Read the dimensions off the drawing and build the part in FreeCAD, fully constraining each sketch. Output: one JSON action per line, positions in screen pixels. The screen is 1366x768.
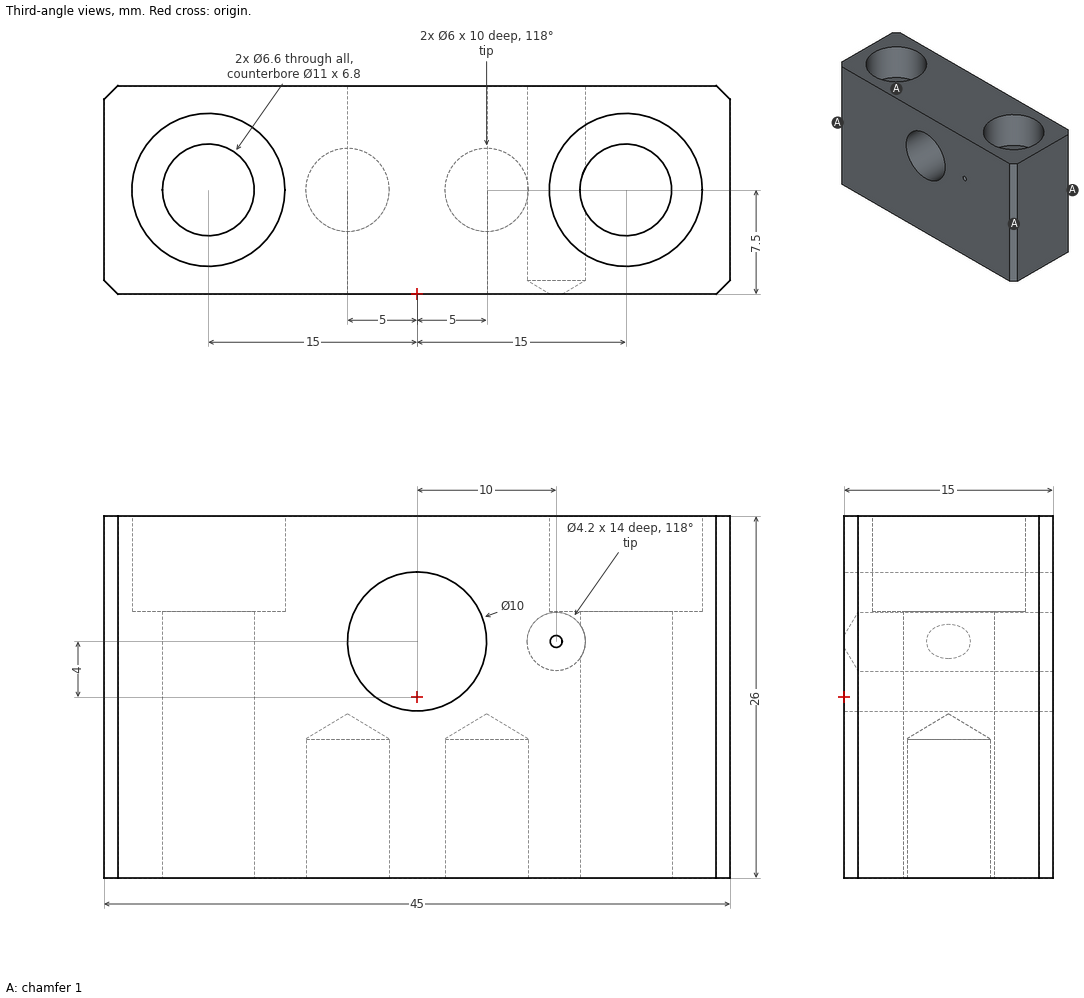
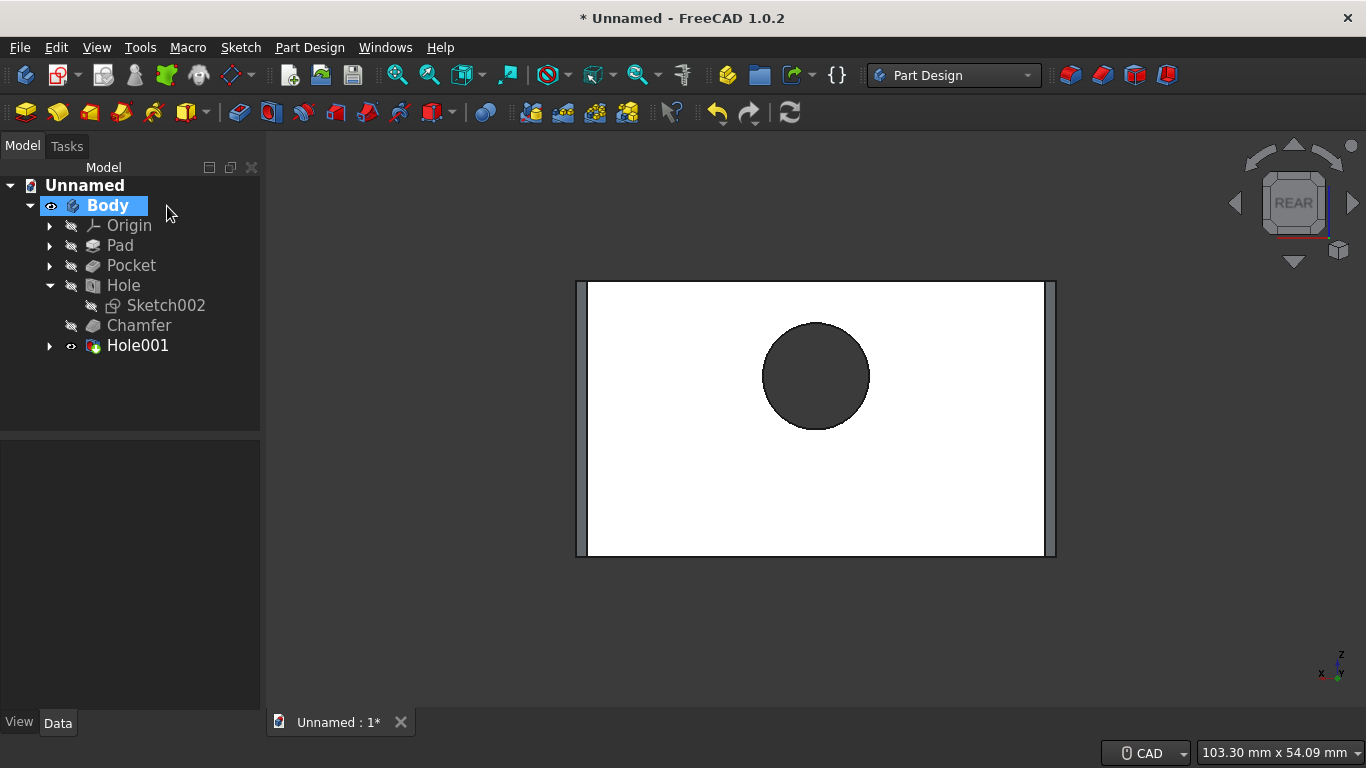
{"action": "left_click", "coordinate": [685, 458]}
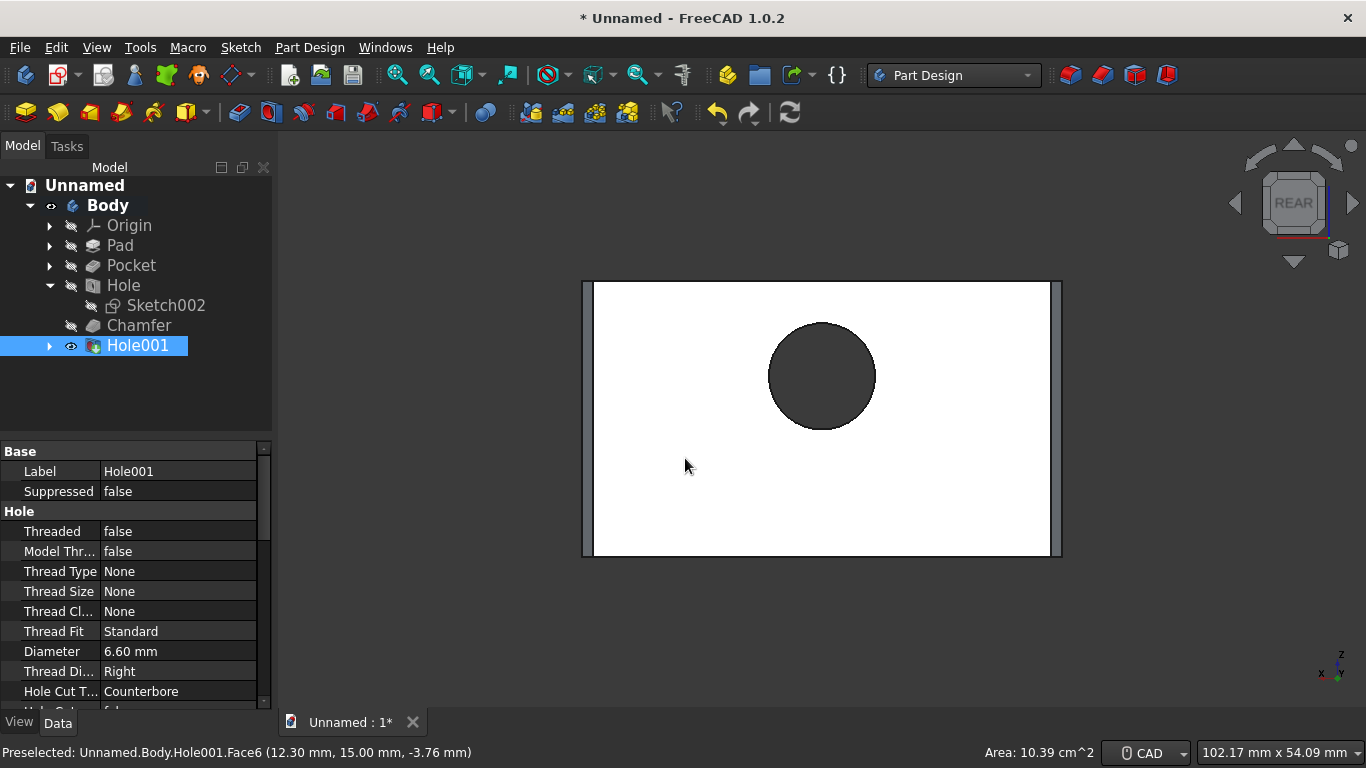
{"action": "left_click", "coordinate": [58, 76]}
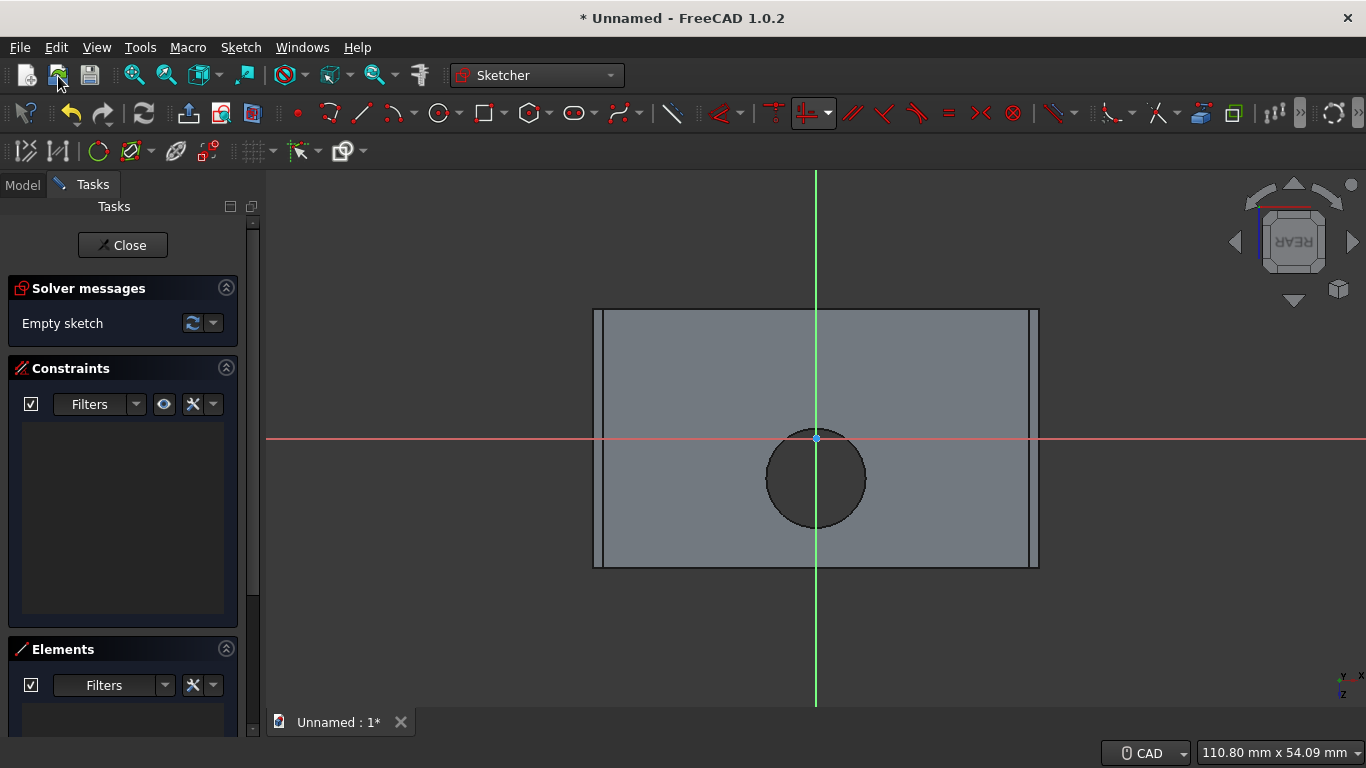
{"action": "scroll", "coordinate": [942, 484], "scroll_direction": "up", "scroll_amount": 10}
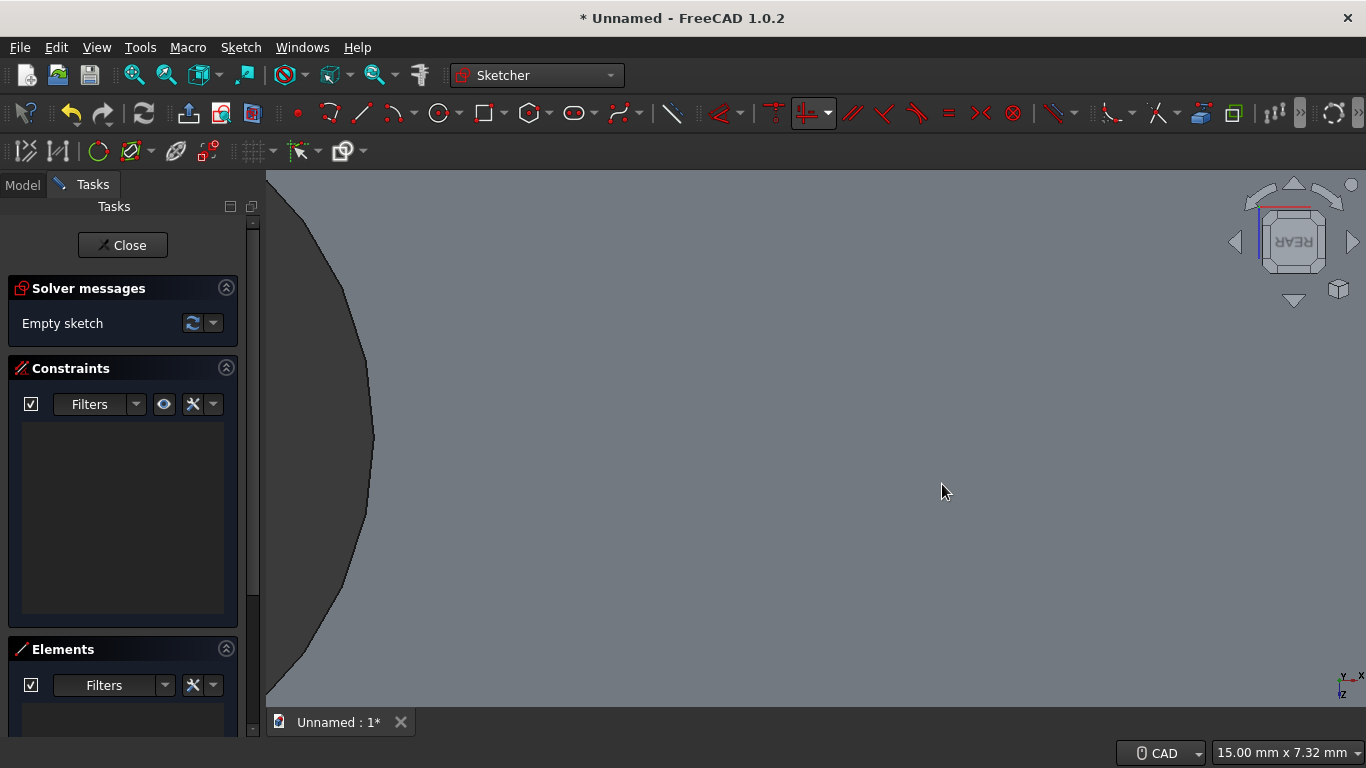
{"action": "left_click", "coordinate": [440, 114]}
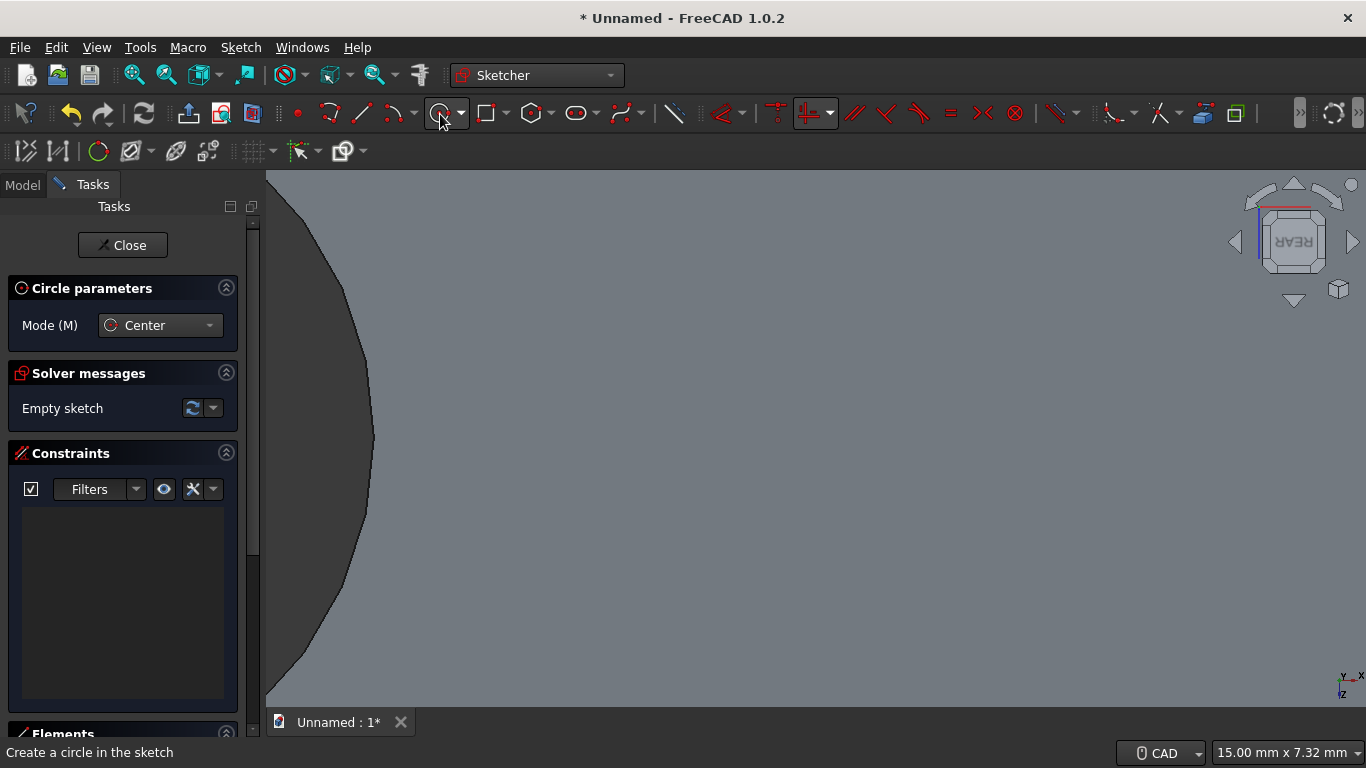
{"action": "left_click", "coordinate": [741, 437]}
{"action": "left_click", "coordinate": [850, 329]}
{"action": "key", "text": "Escape"}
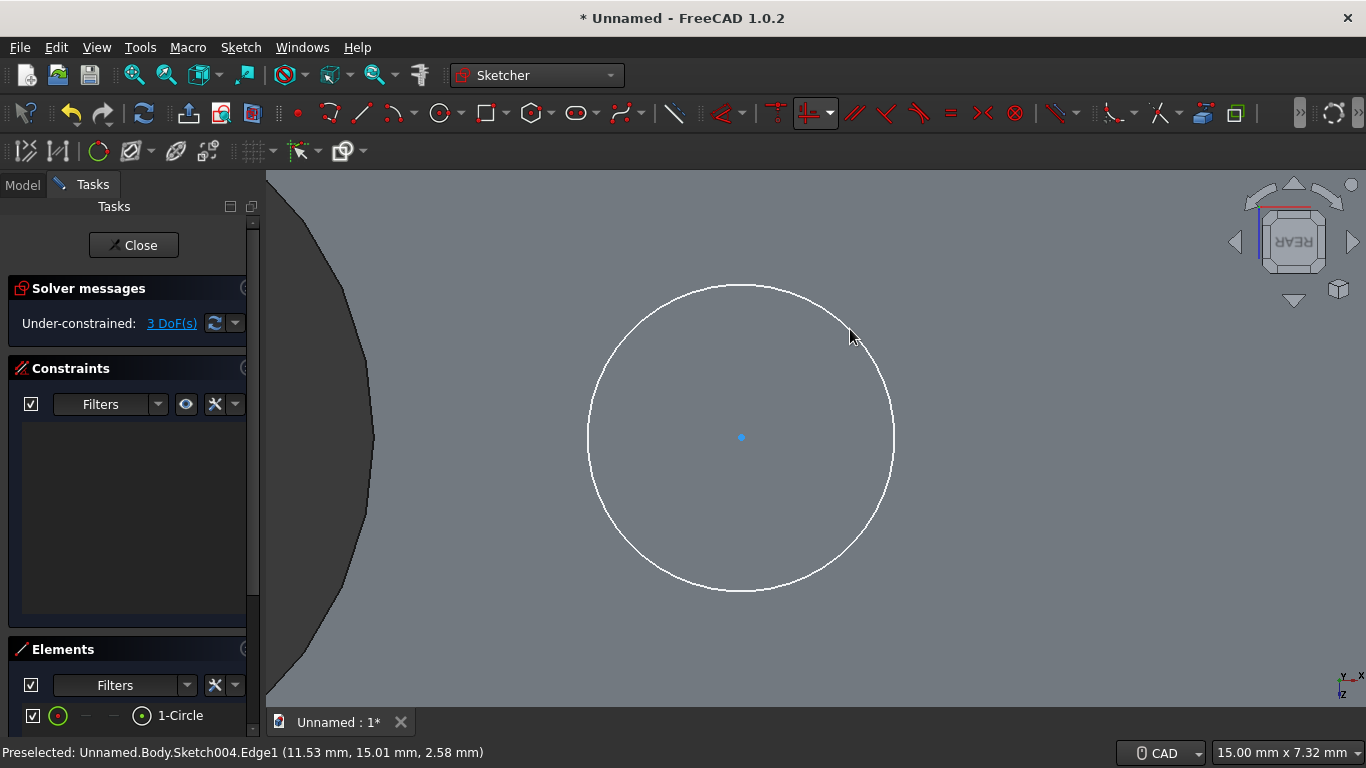
{"action": "left_click", "coordinate": [722, 114]}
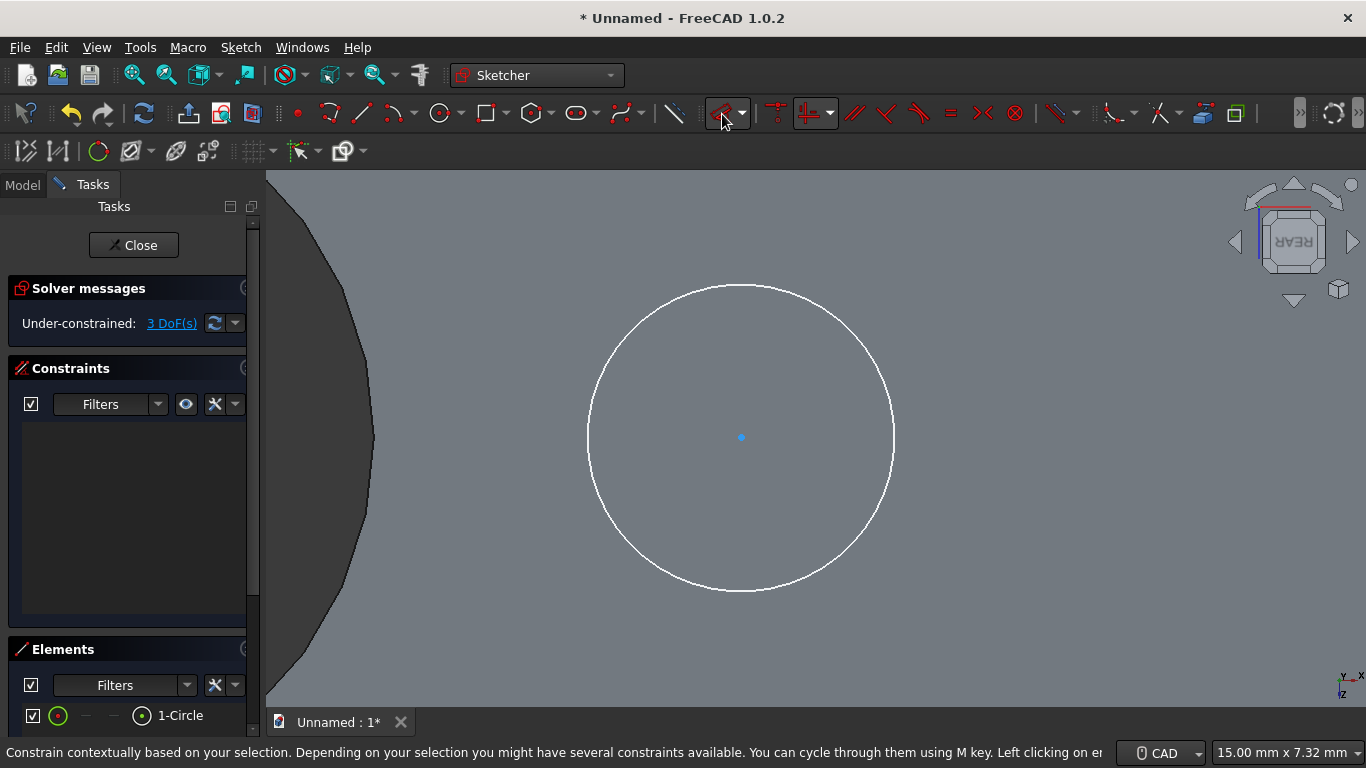
{"action": "left_click", "coordinate": [849, 329]}
{"action": "left_click", "coordinate": [872, 306]}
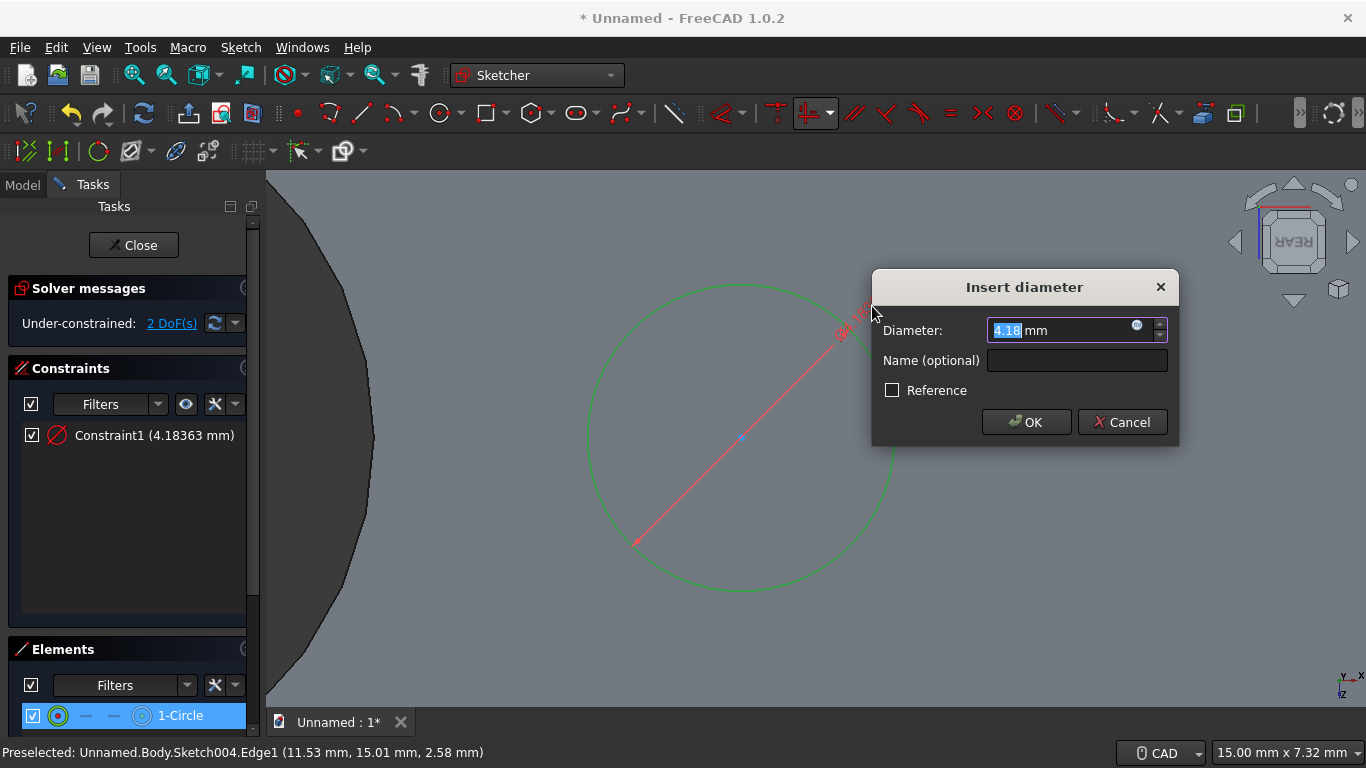
{"action": "type", "text": "4.2"}
{"action": "key", "text": "Return"}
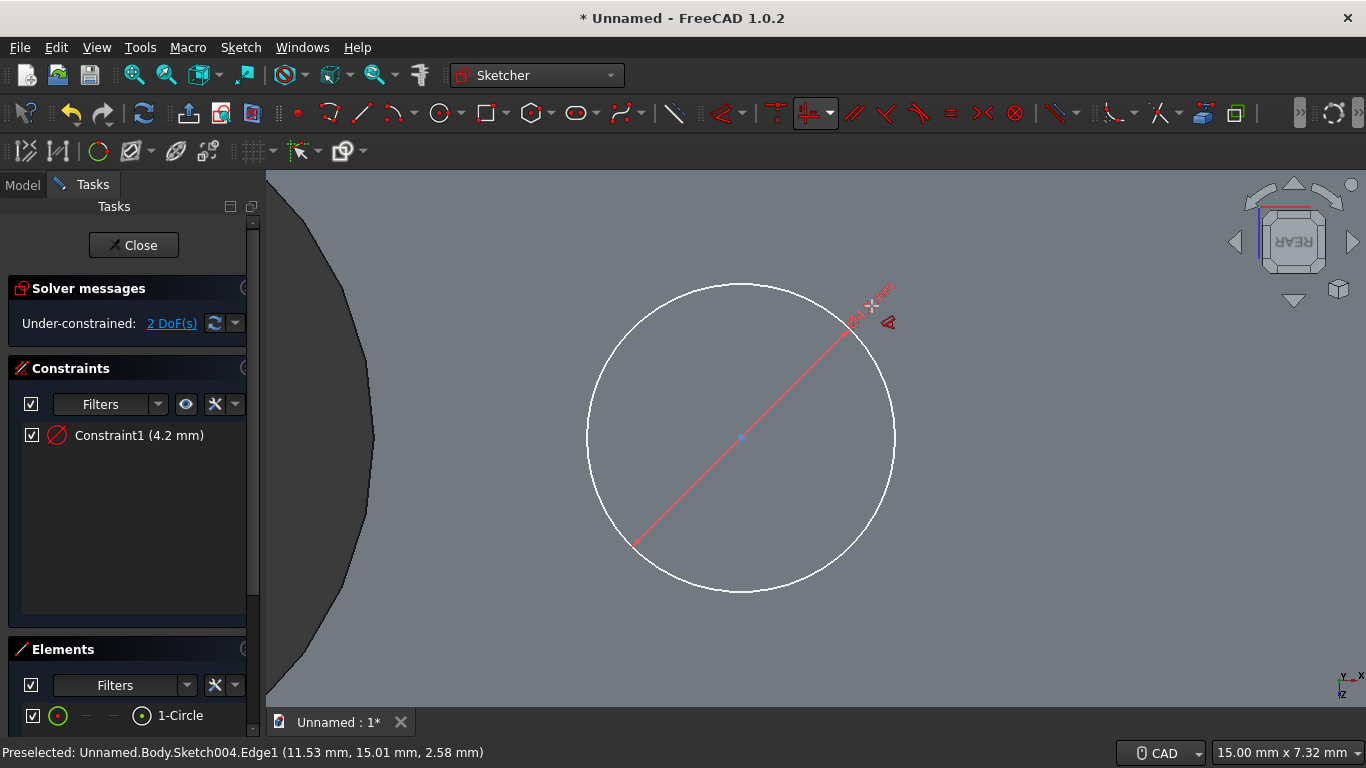
{"action": "left_click", "coordinate": [741, 438]}
{"action": "left_click", "coordinate": [775, 318]}